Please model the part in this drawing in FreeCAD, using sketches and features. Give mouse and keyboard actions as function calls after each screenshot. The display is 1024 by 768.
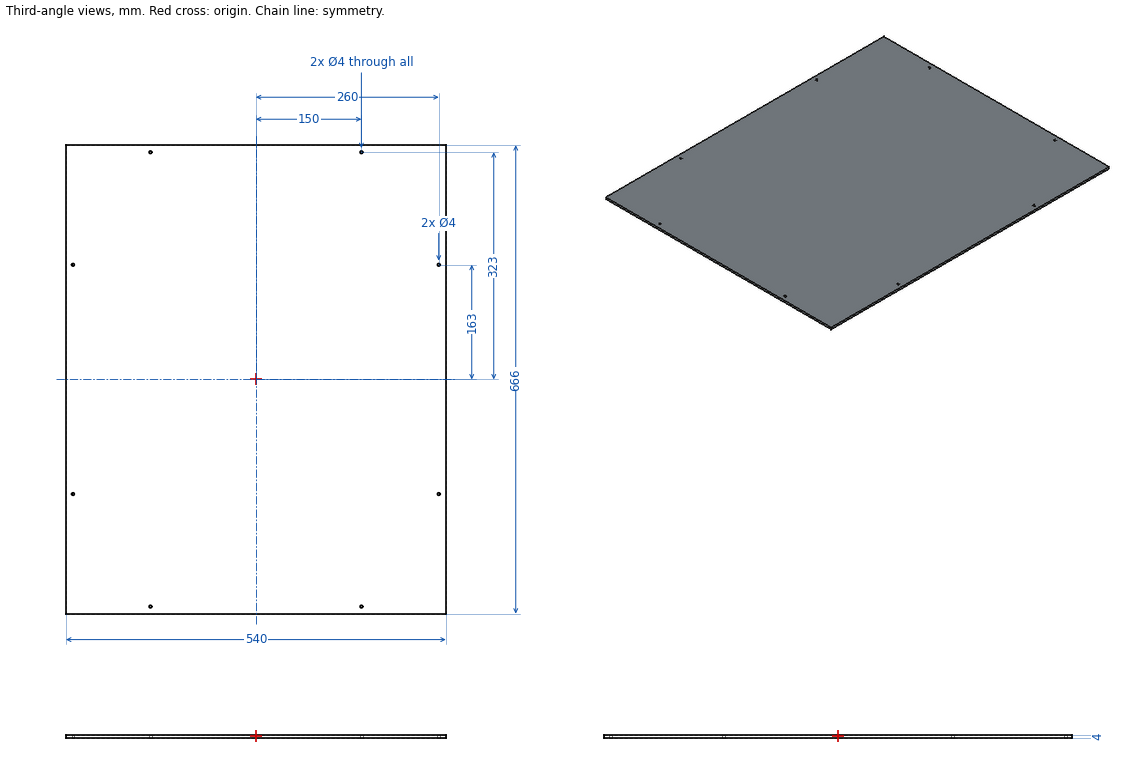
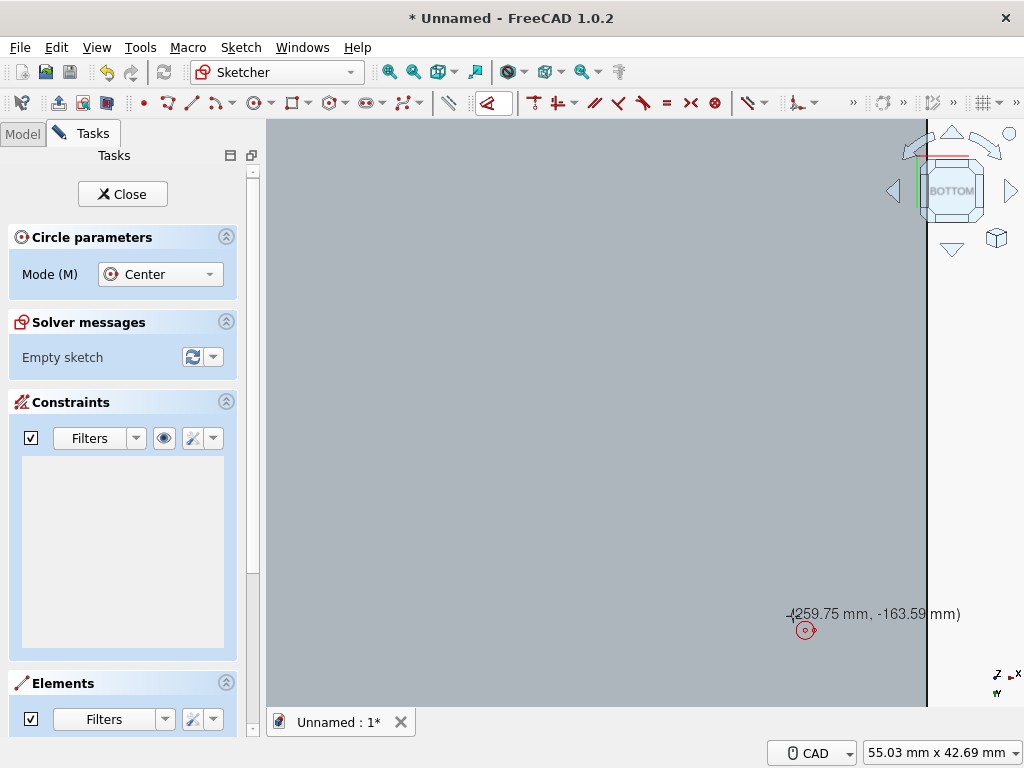
scroll(733, 617, down, 12)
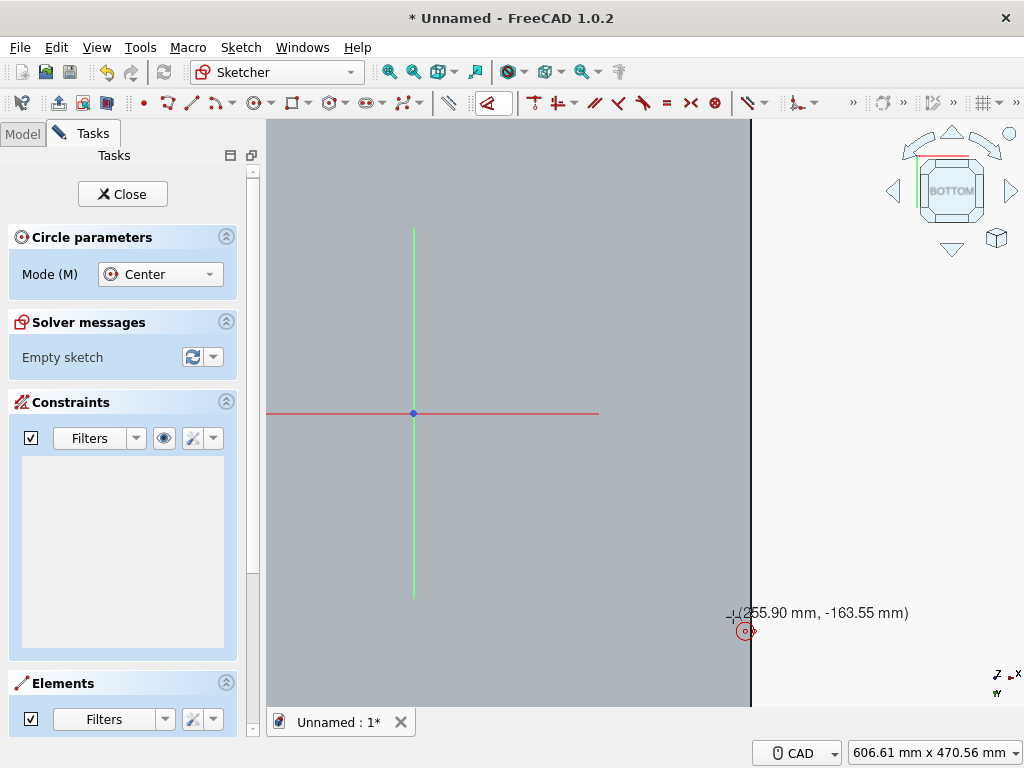
click(739, 617)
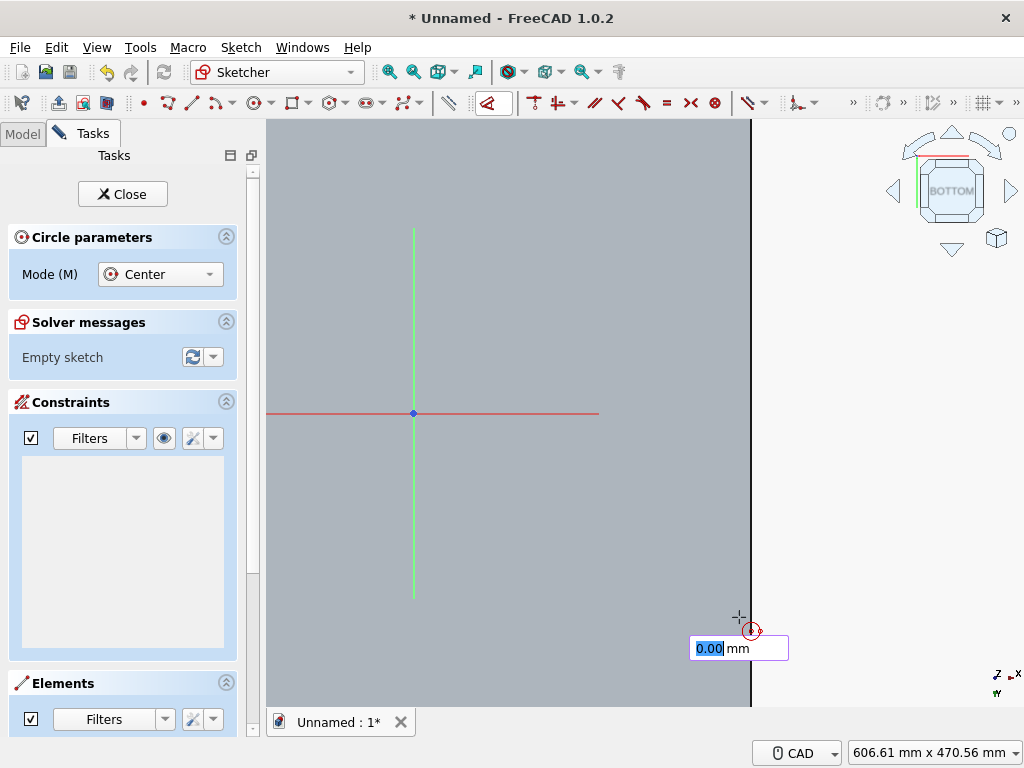
scroll(740, 615, up, 10)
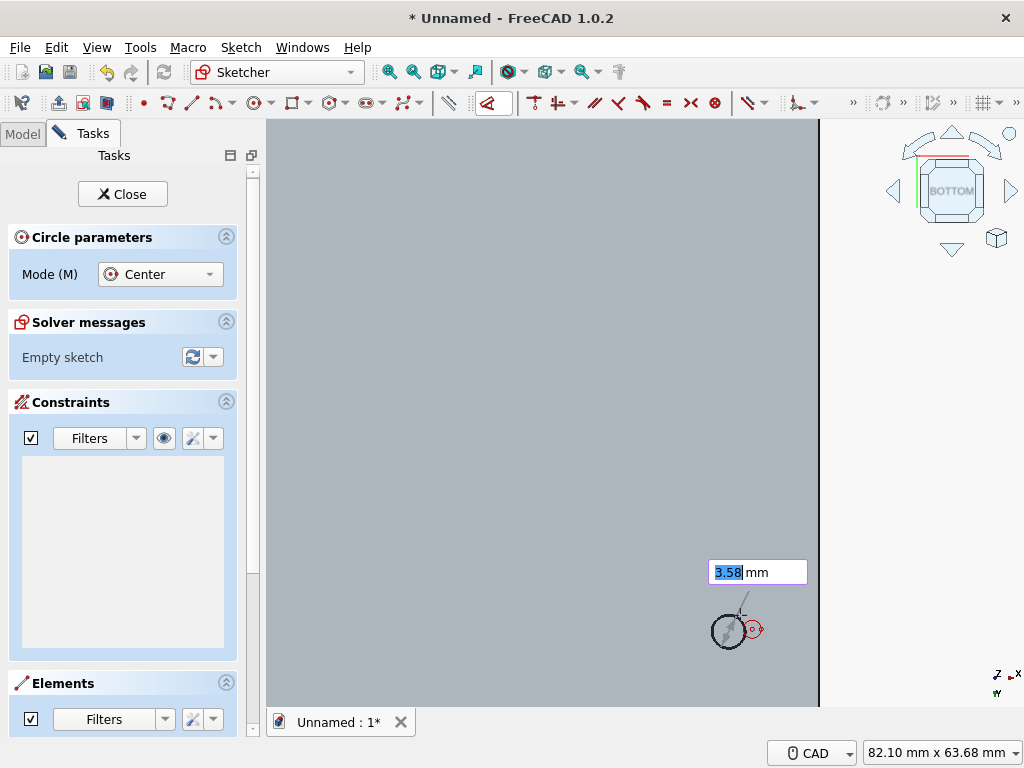
click(739, 613)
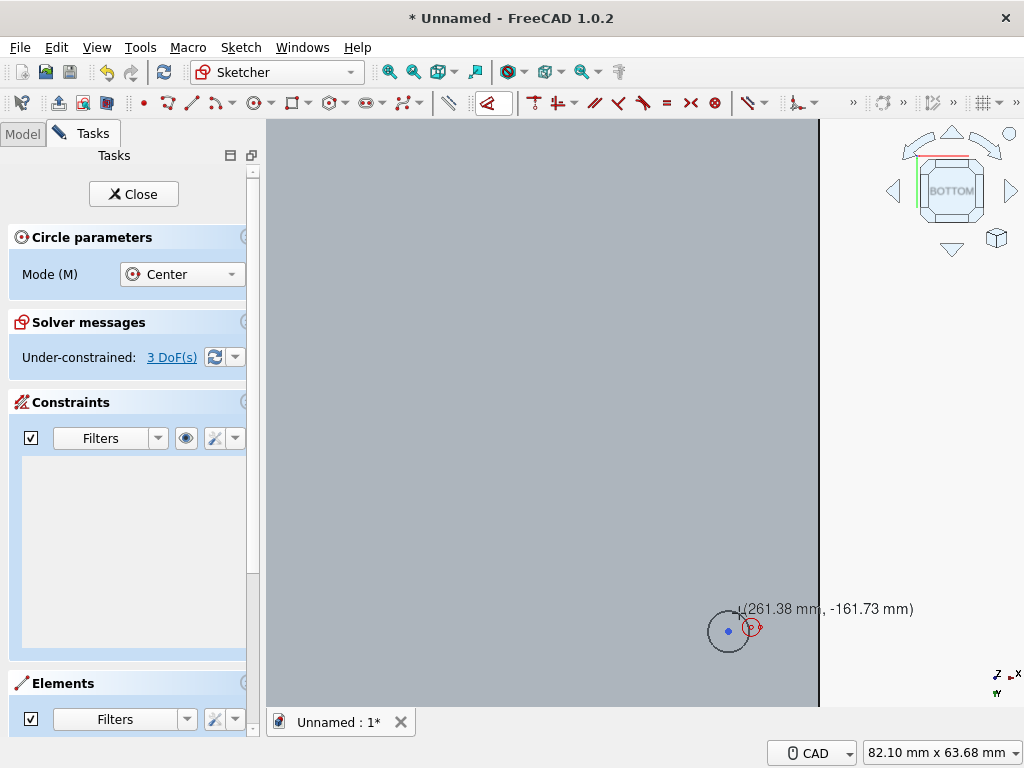
scroll(739, 615, down, 10)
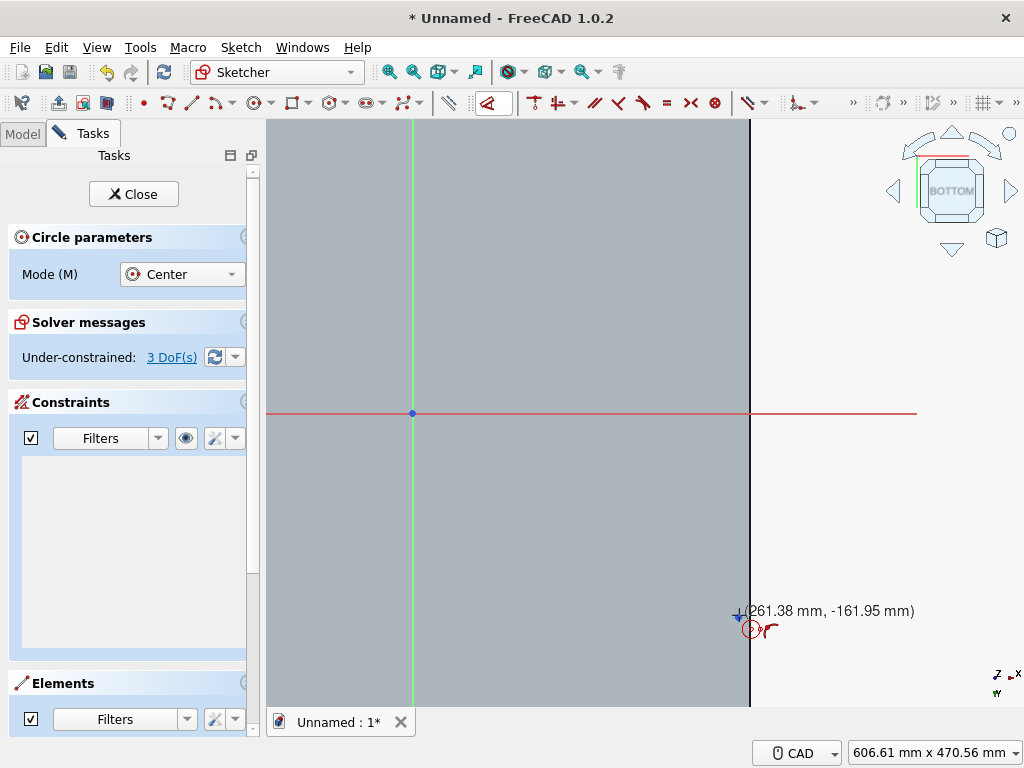
scroll(738, 210, up, 12)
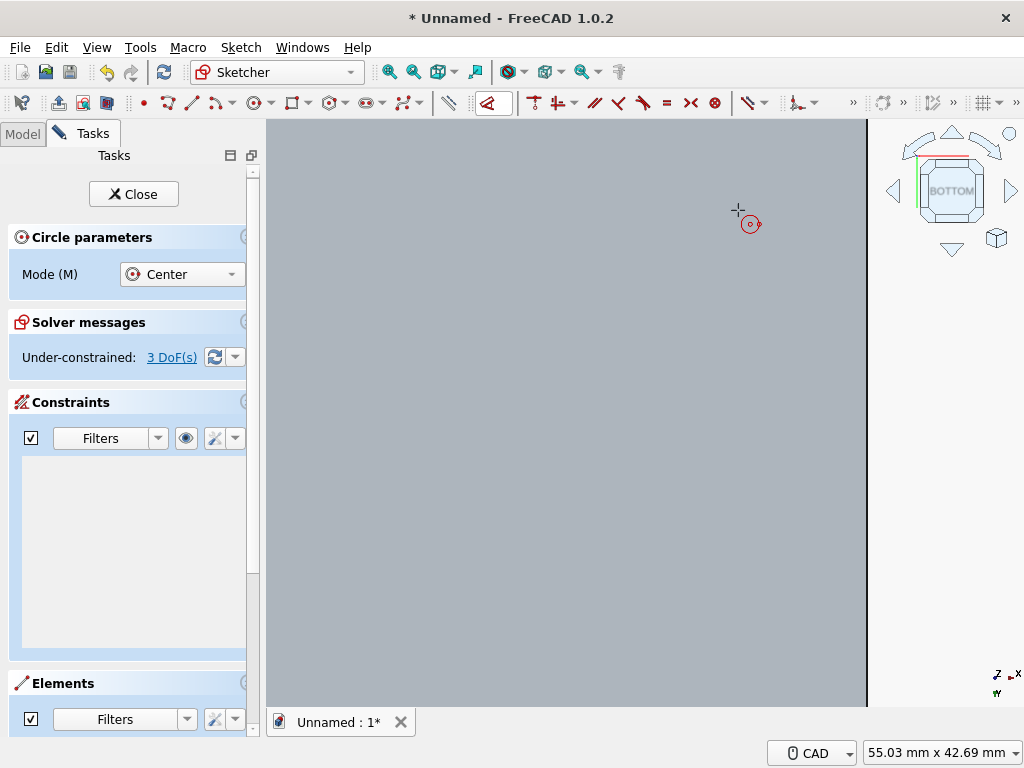
scroll(738, 210, down, 12)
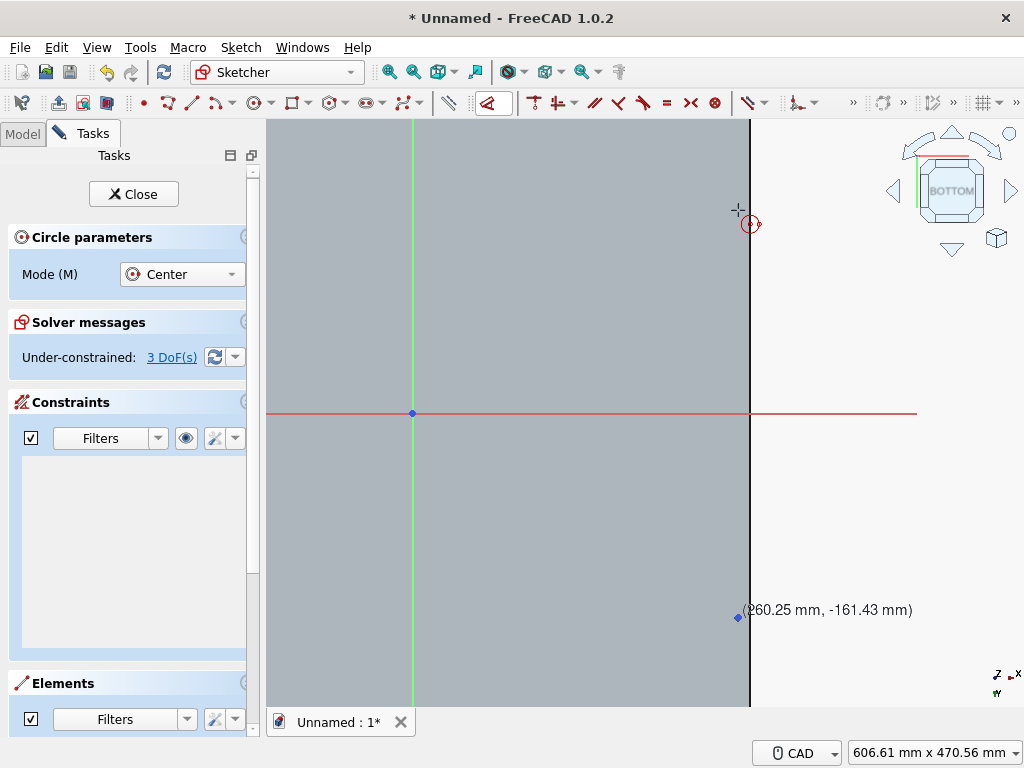
click(738, 210)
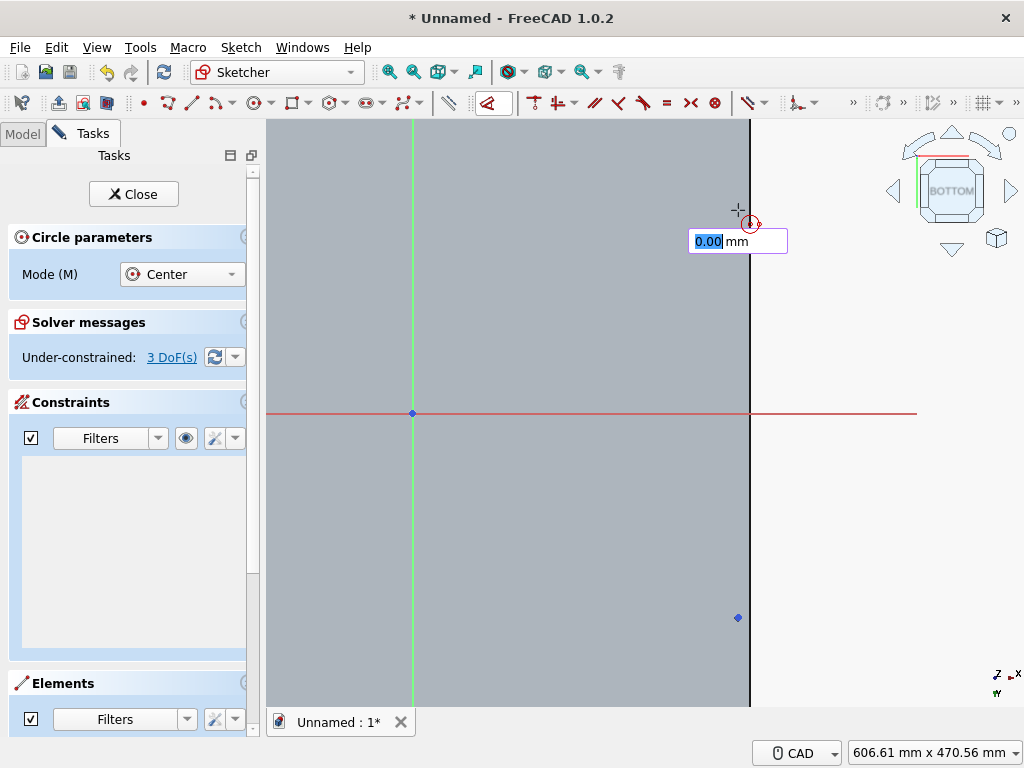
scroll(740, 208, up, 10)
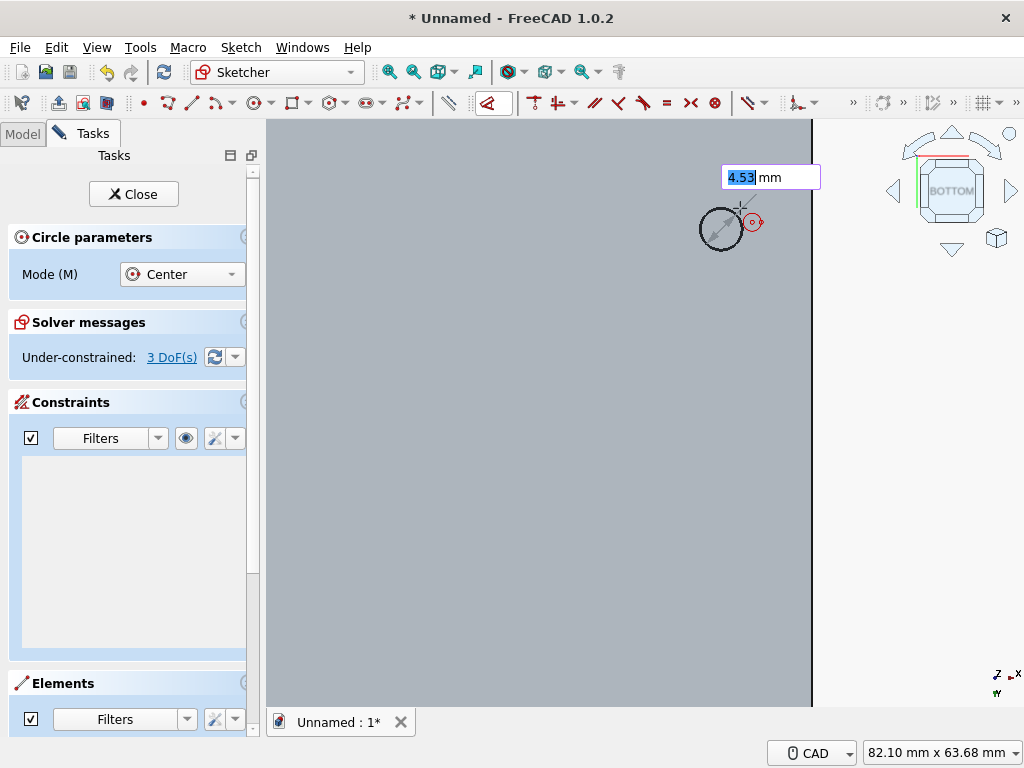
click(733, 207)
key(Escape)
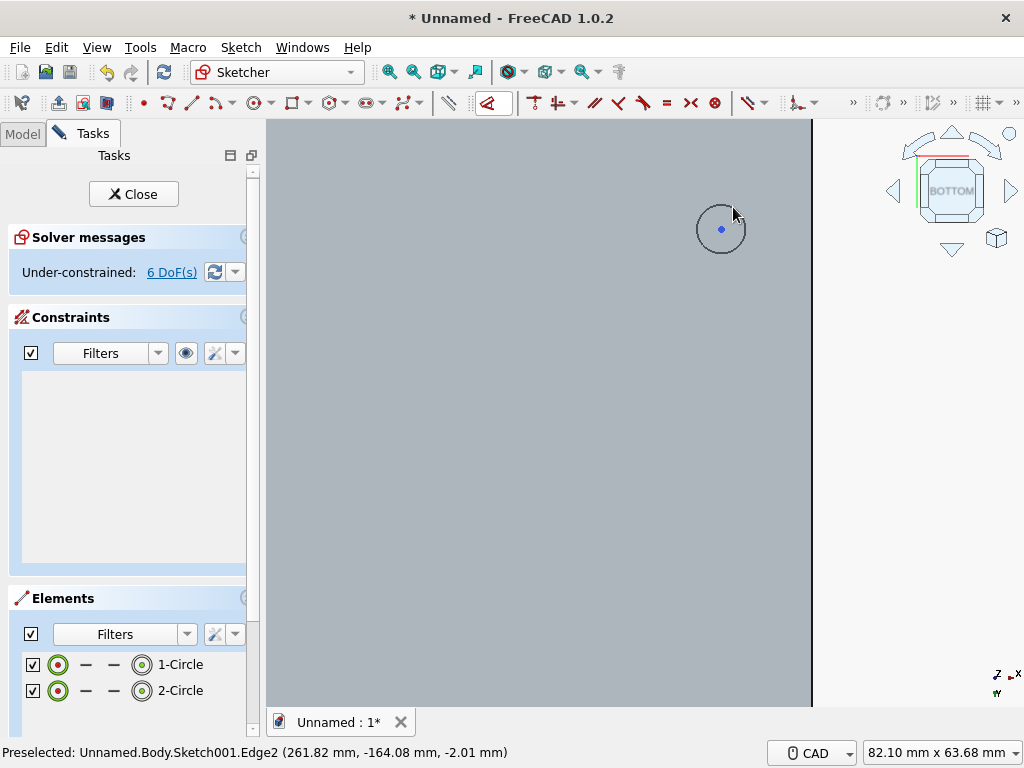
scroll(740, 208, down, 10)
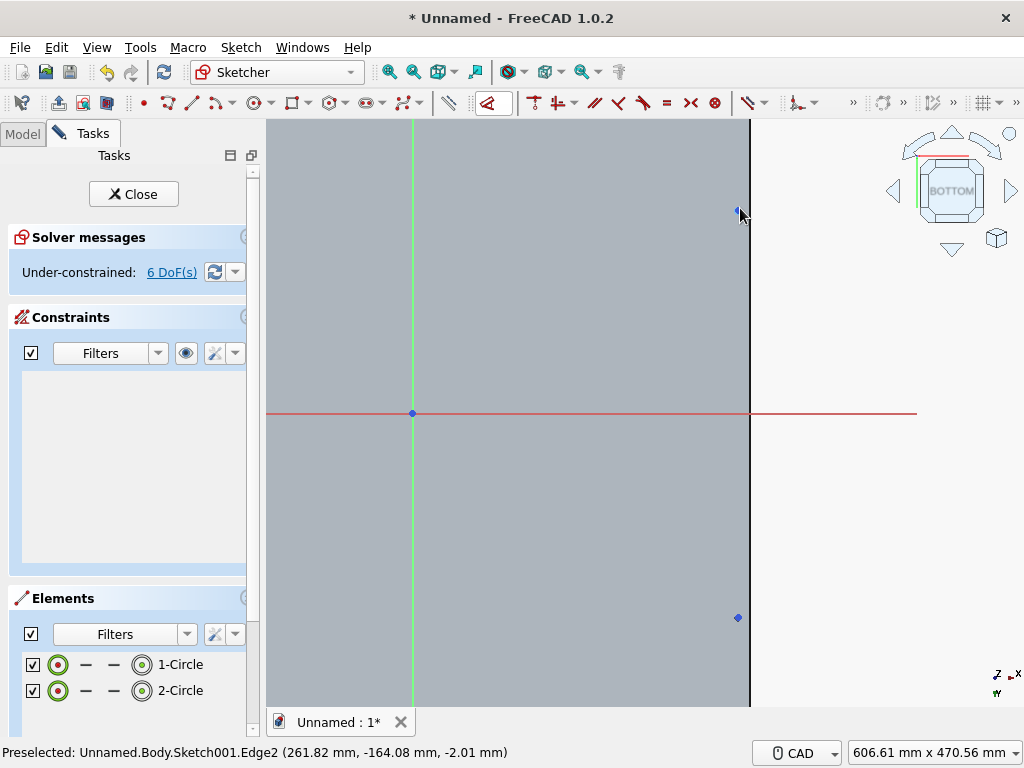
scroll(740, 616, up, 9)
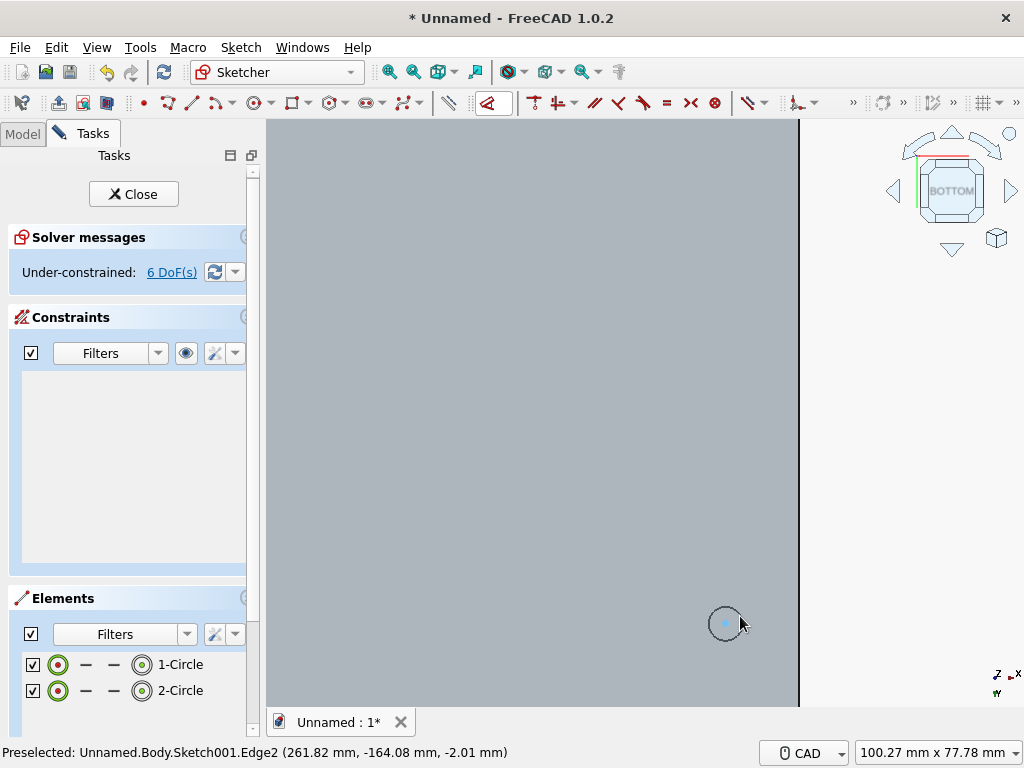
click(737, 612)